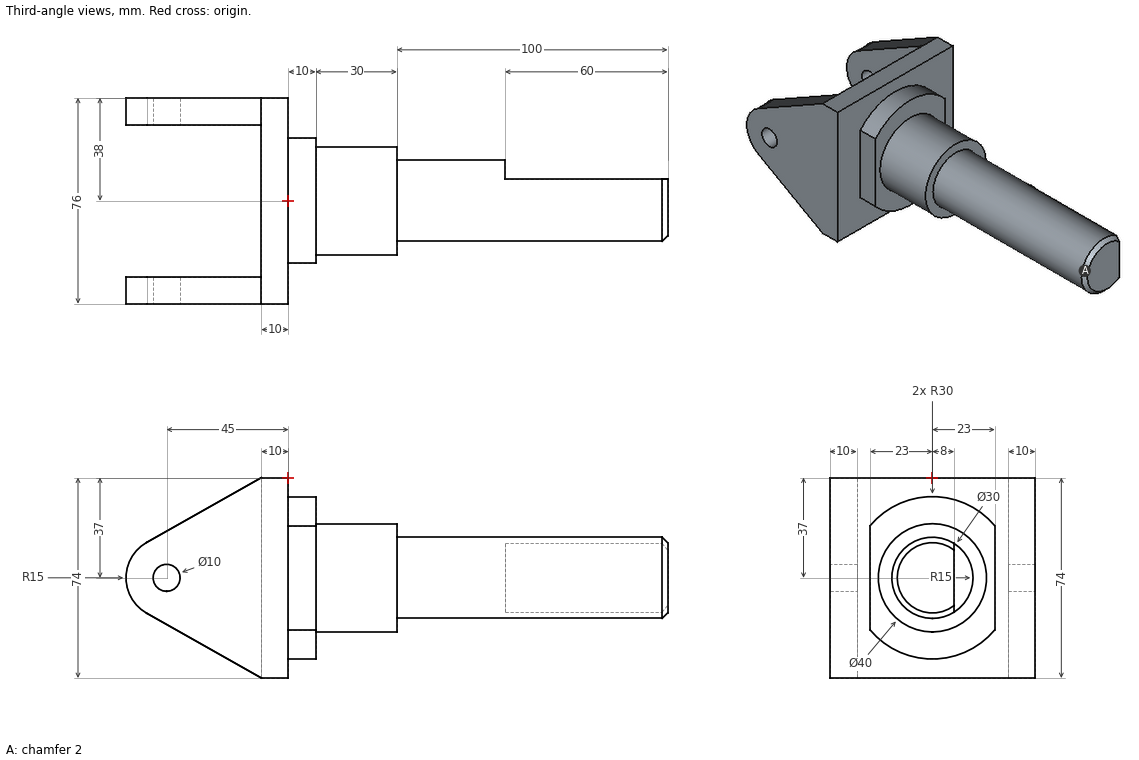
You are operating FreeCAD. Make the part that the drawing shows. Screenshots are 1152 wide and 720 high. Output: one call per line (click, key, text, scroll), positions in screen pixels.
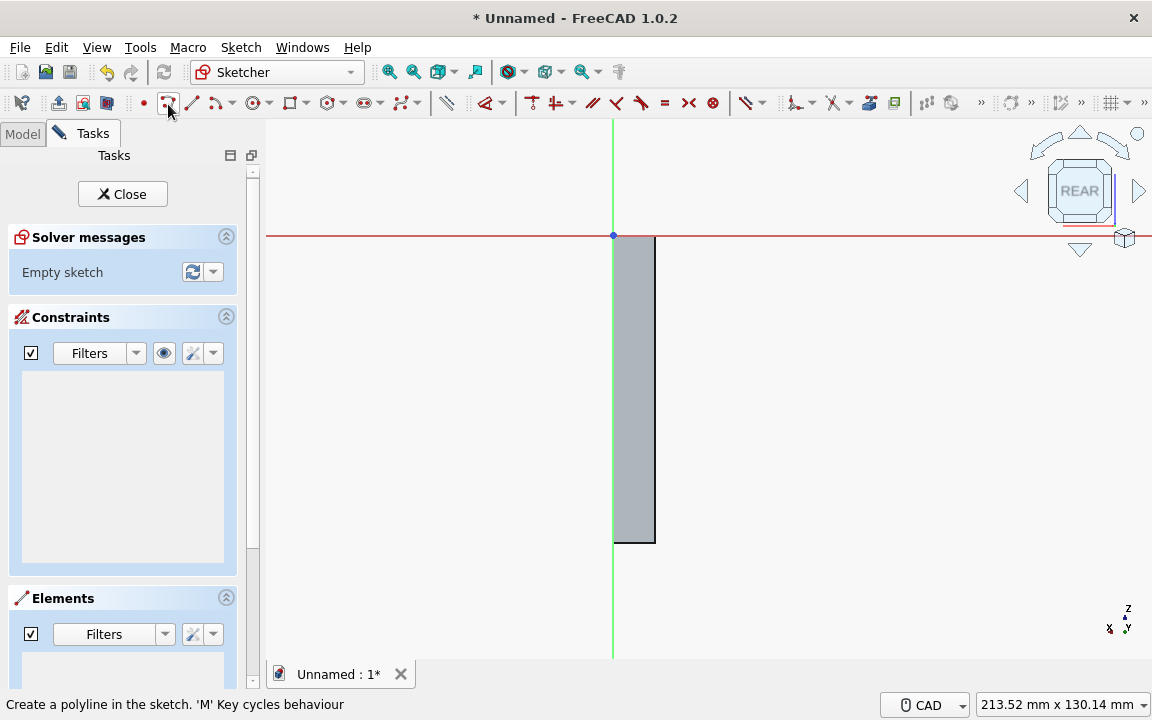
click(830, 335)
click(655, 236)
click(655, 543)
click(830, 443)
right_click(830, 443)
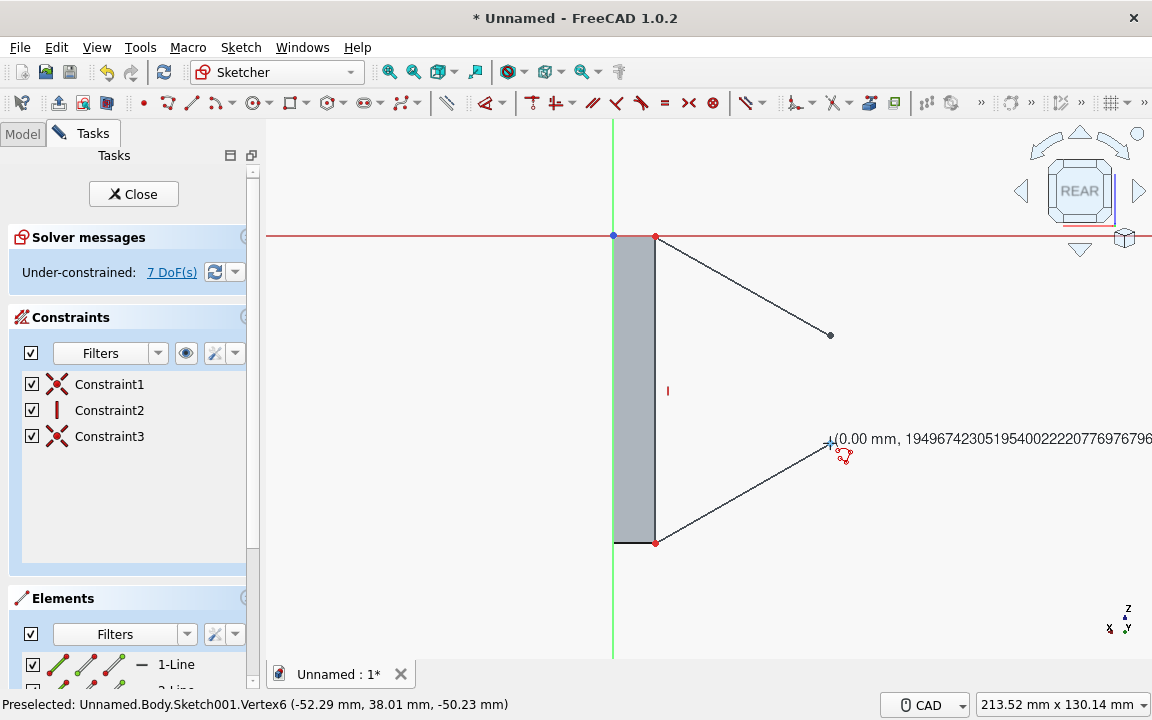
key(g)
key(3)
key(a)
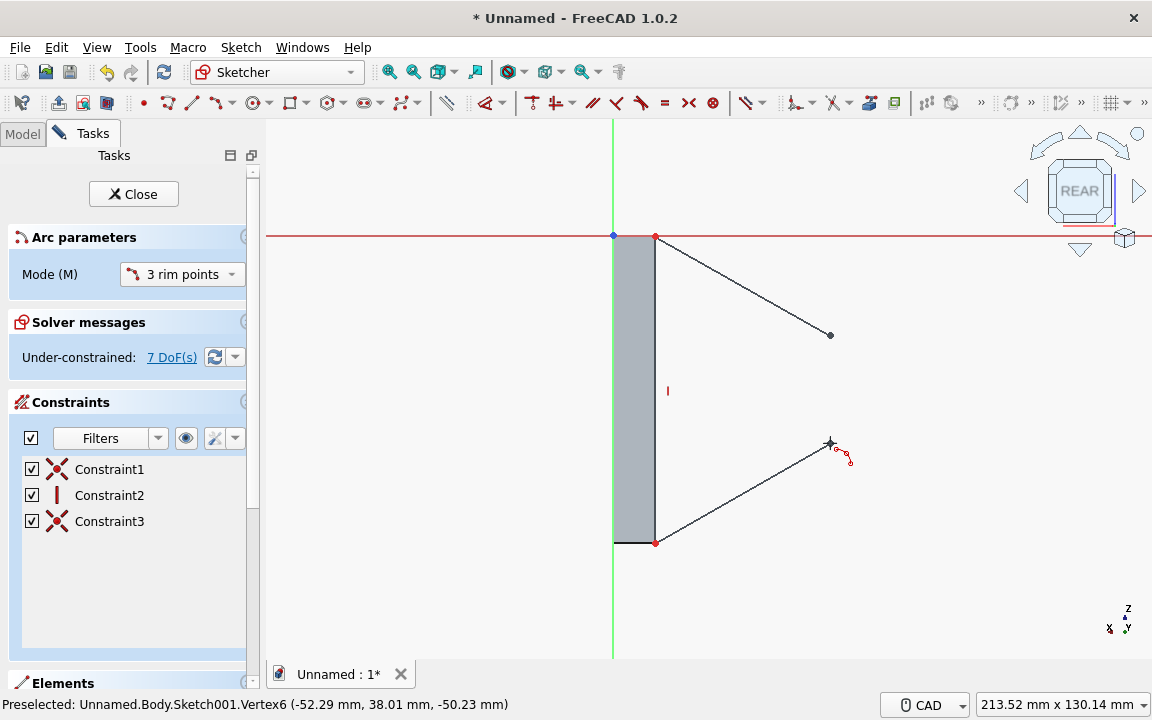
click(830, 444)
click(830, 336)
click(862, 389)
key(Escape)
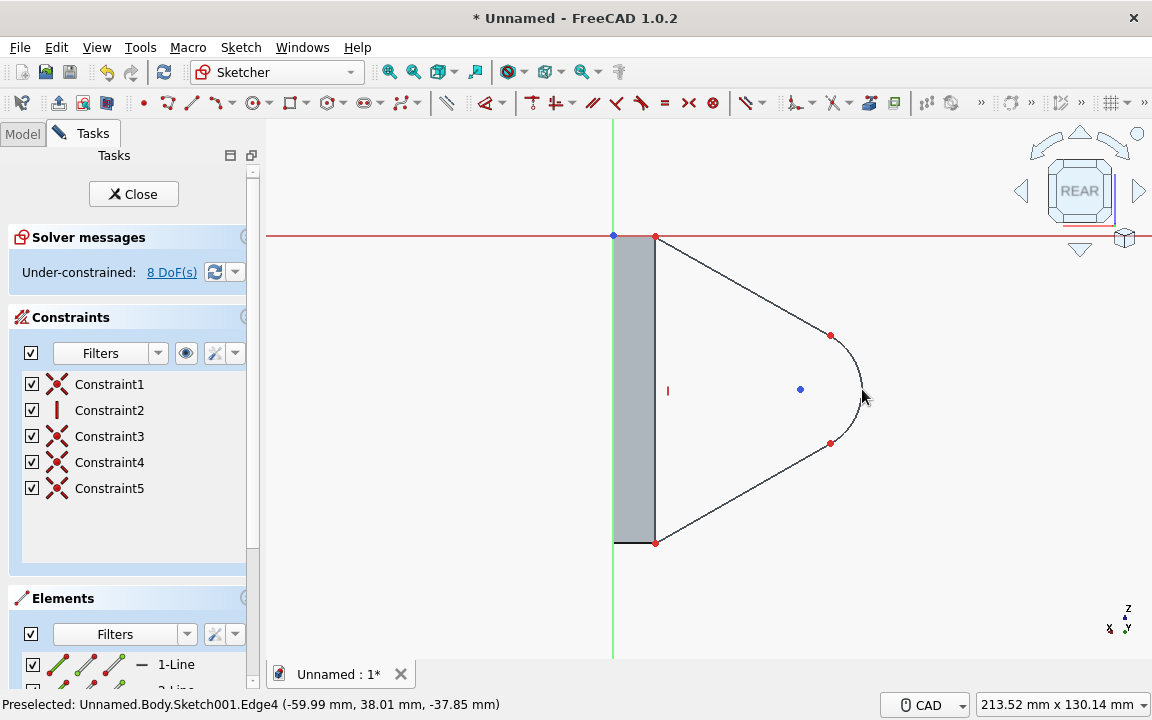
click(777, 306)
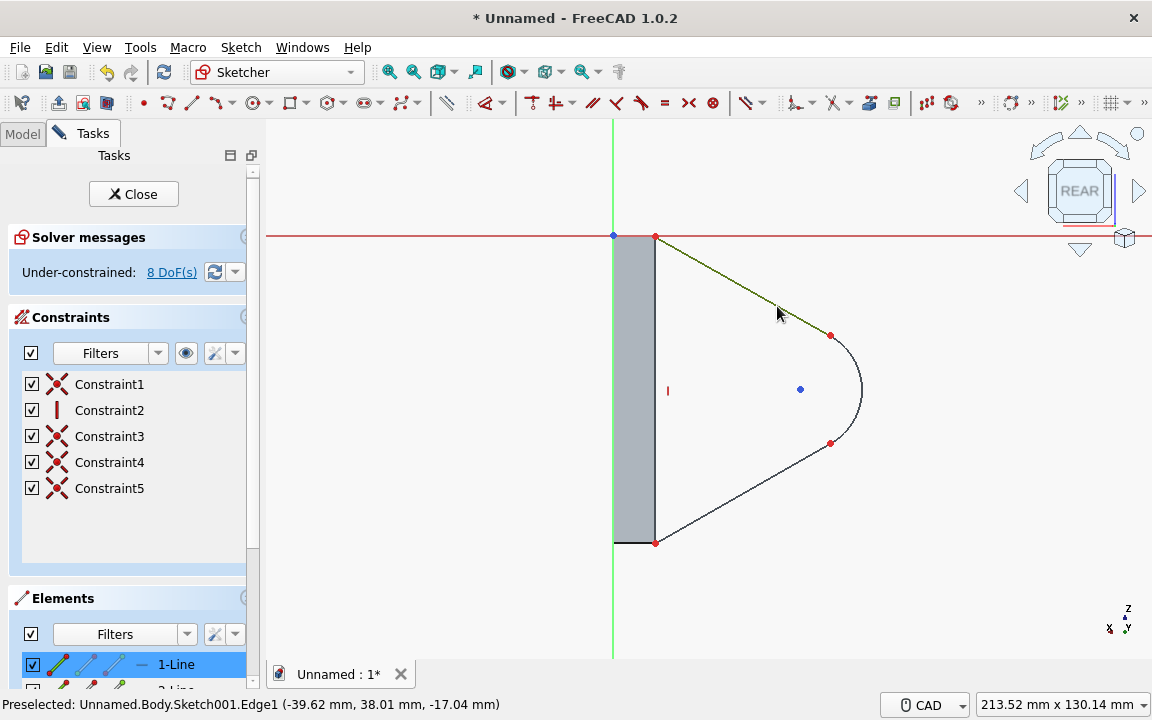
click(856, 416)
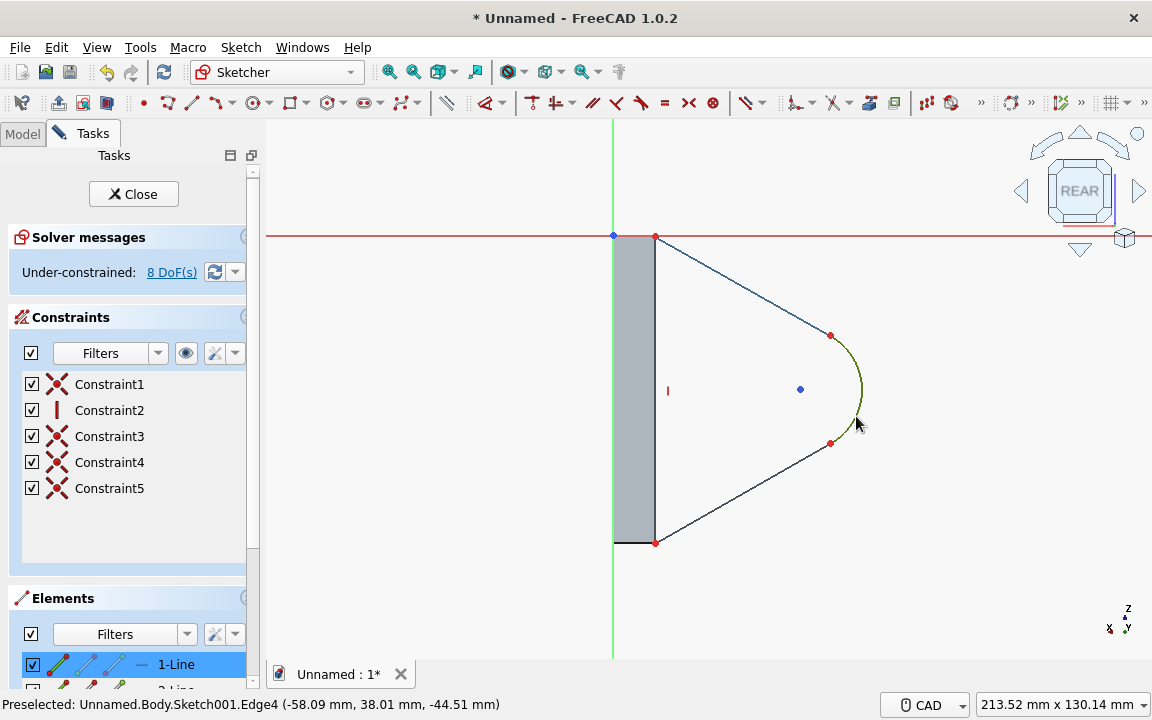
click(642, 104)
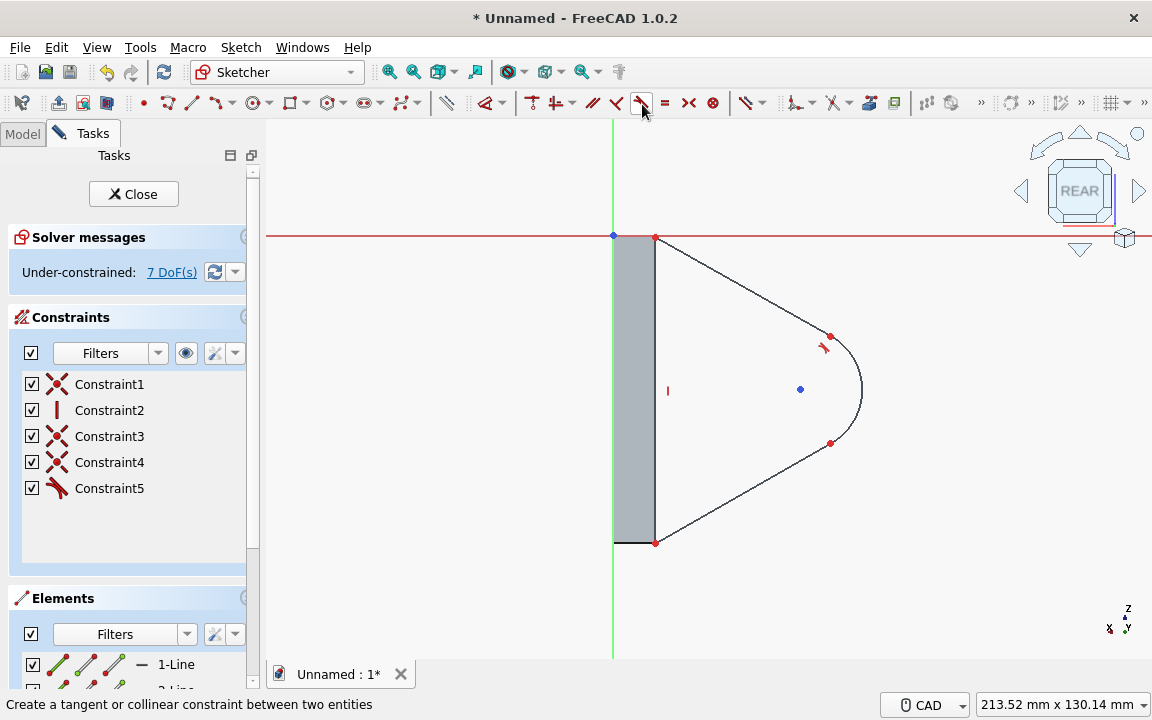
click(707, 514)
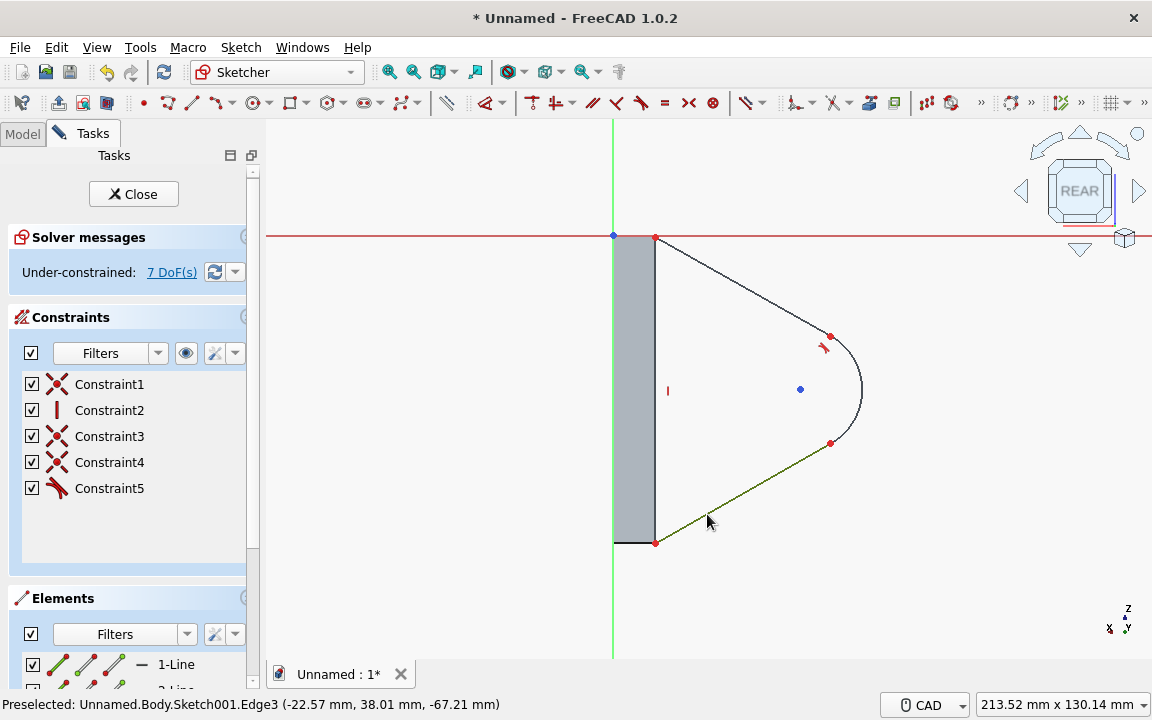
click(856, 416)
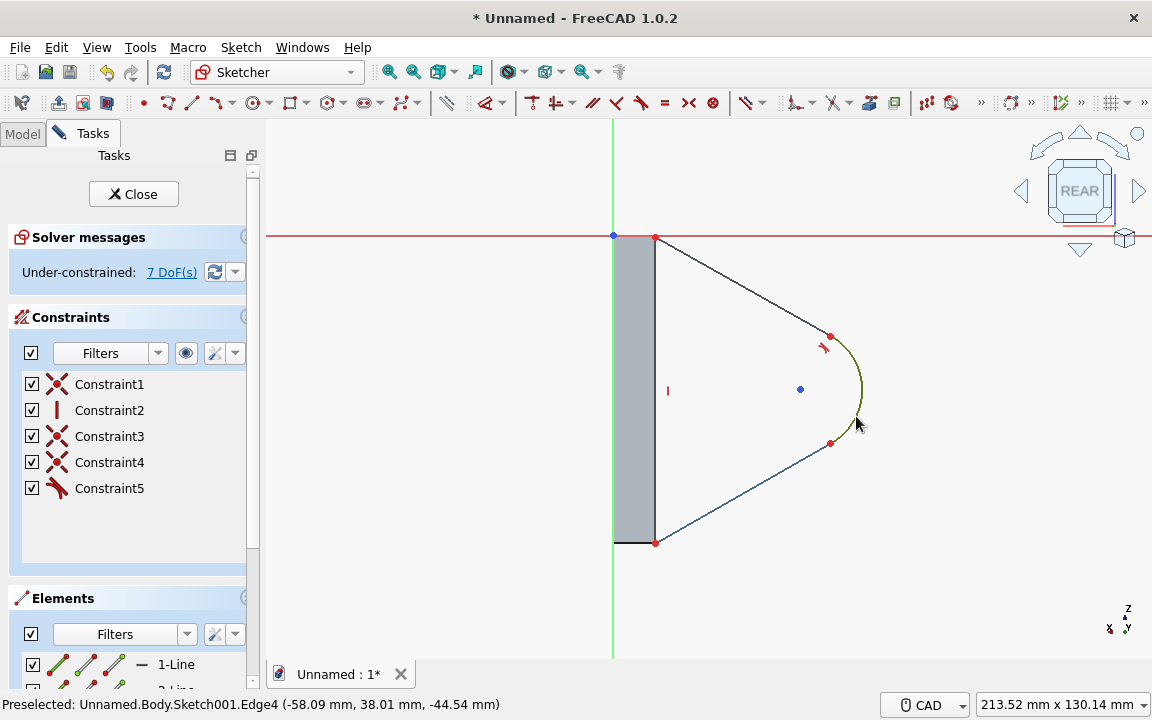
click(642, 104)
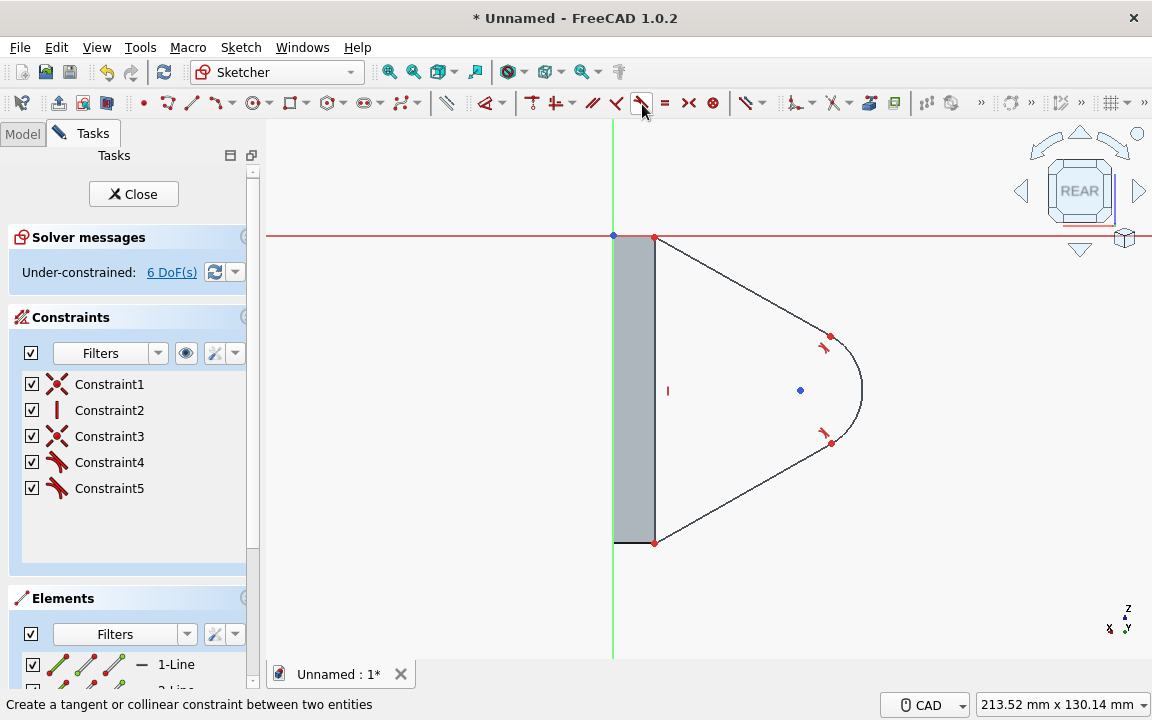
click(486, 104)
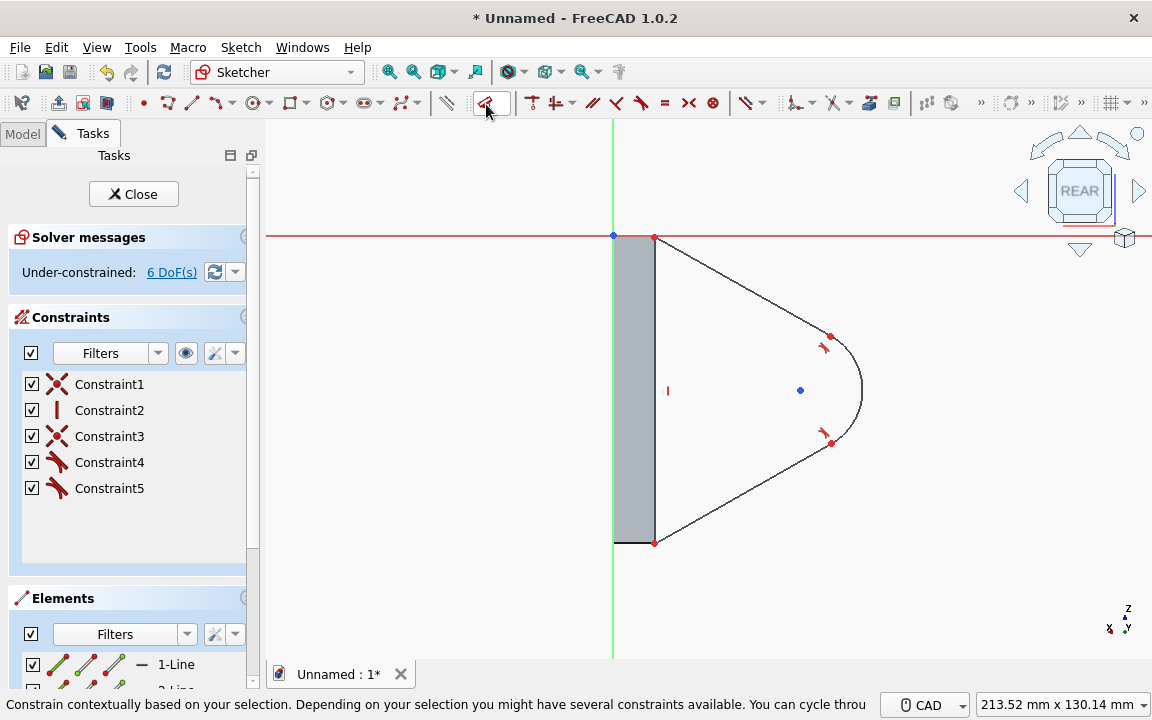
click(857, 415)
click(886, 428)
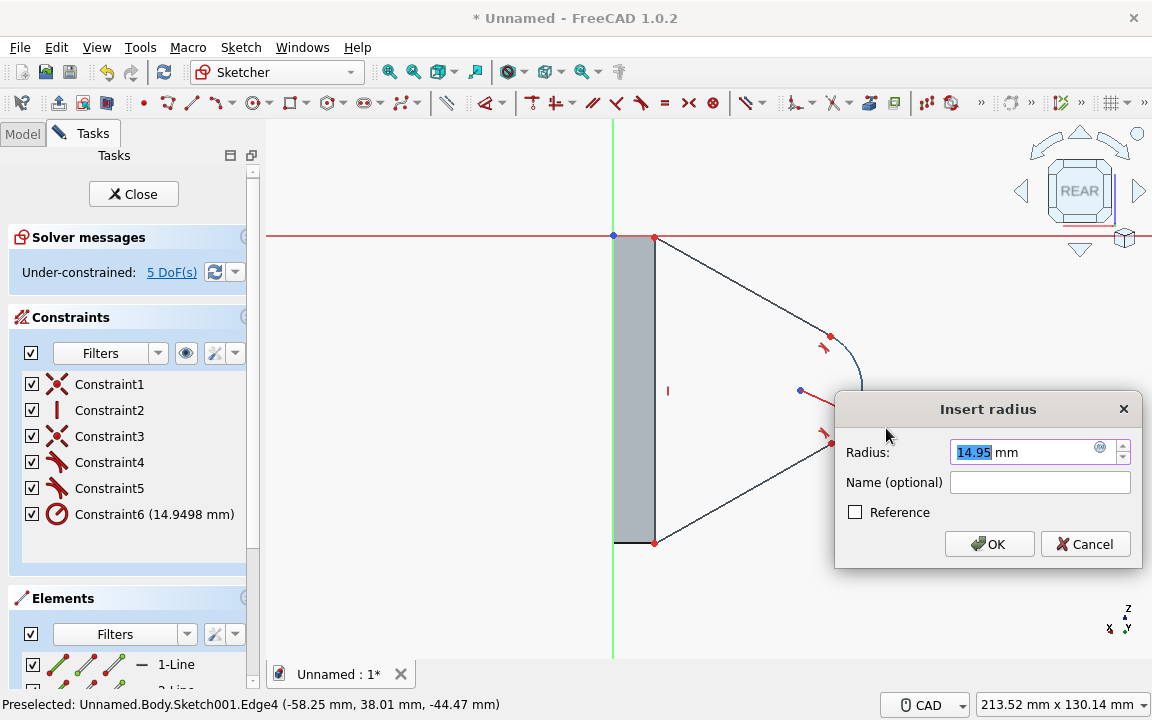
text(15)
key(Return)
key(Escape)